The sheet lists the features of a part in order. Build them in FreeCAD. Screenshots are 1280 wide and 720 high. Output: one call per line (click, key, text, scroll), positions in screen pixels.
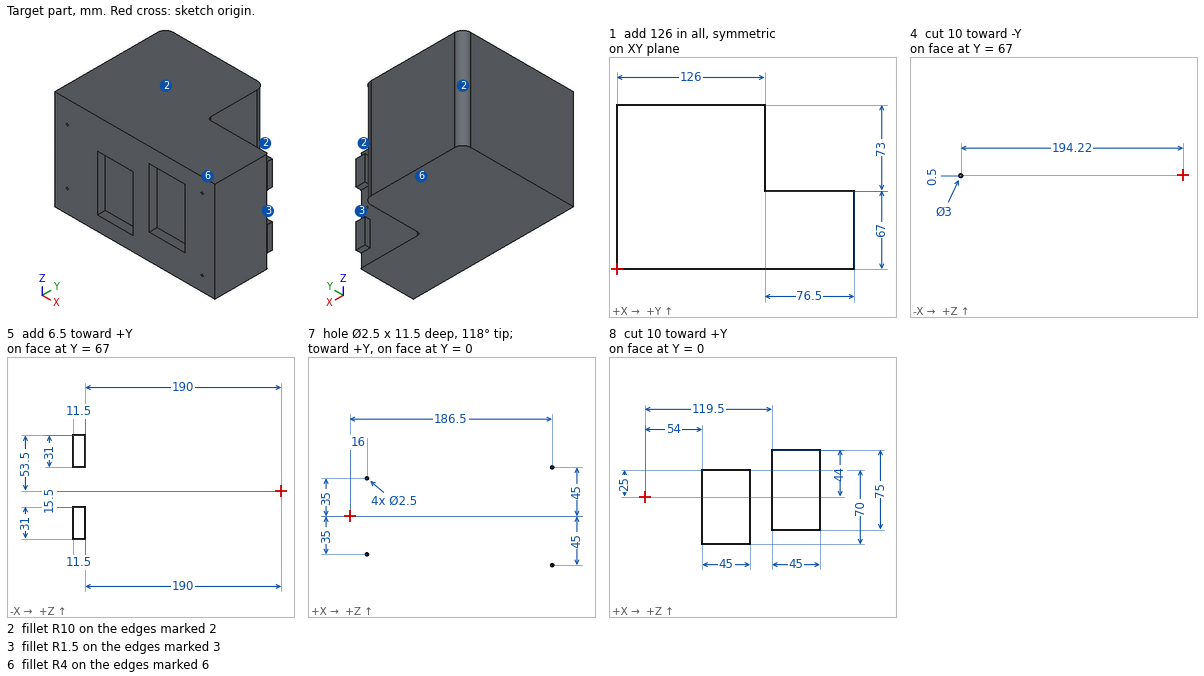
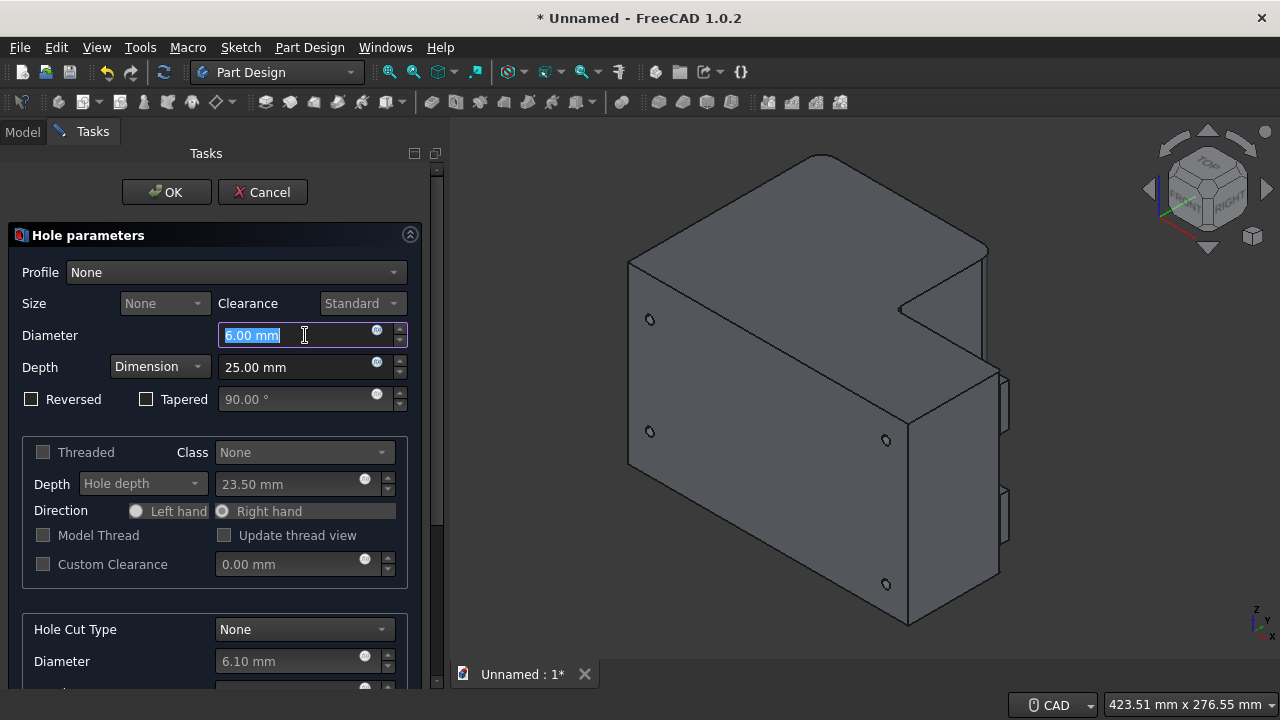
text(2.5)
key(Tab)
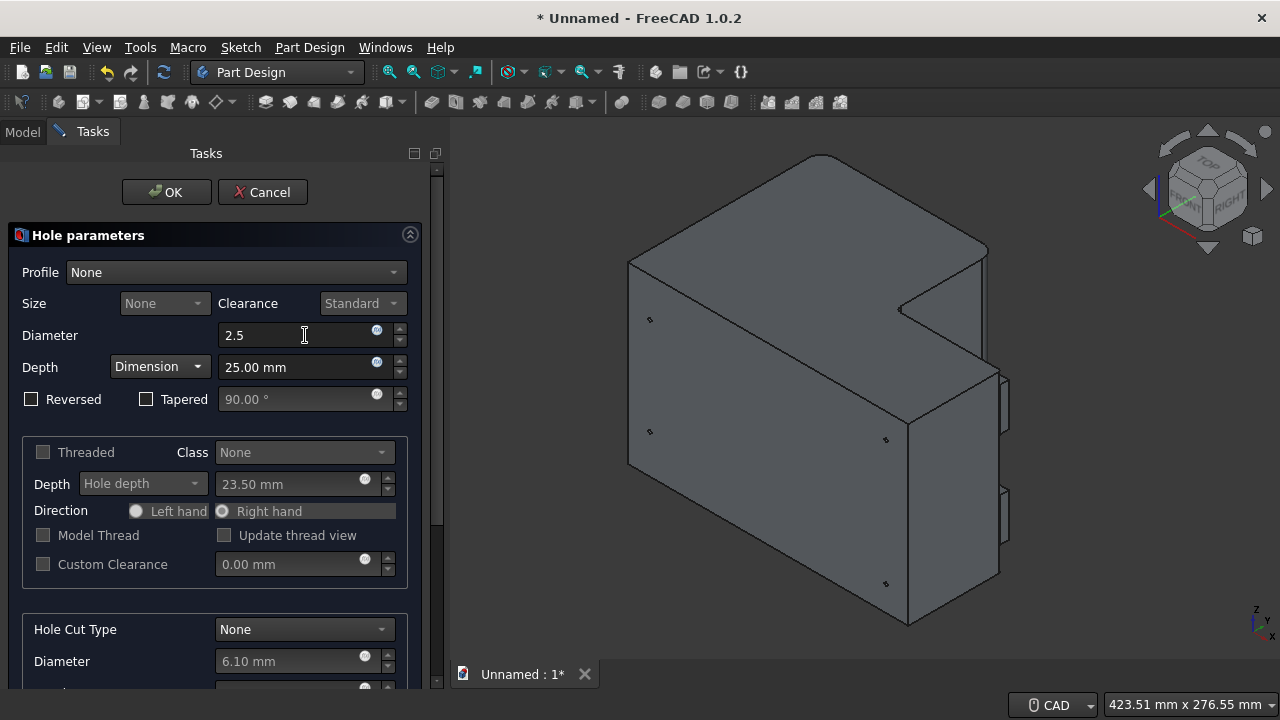
triple_click(305, 367)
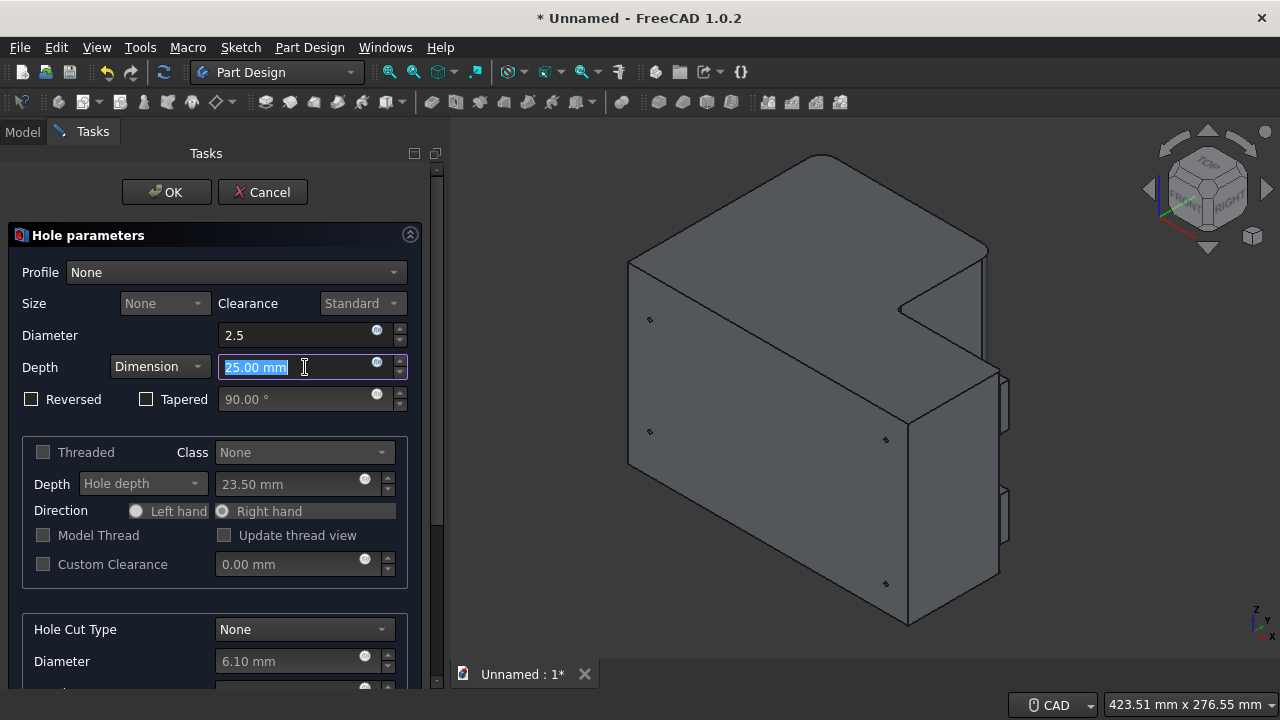
text(11.5)
key(Tab)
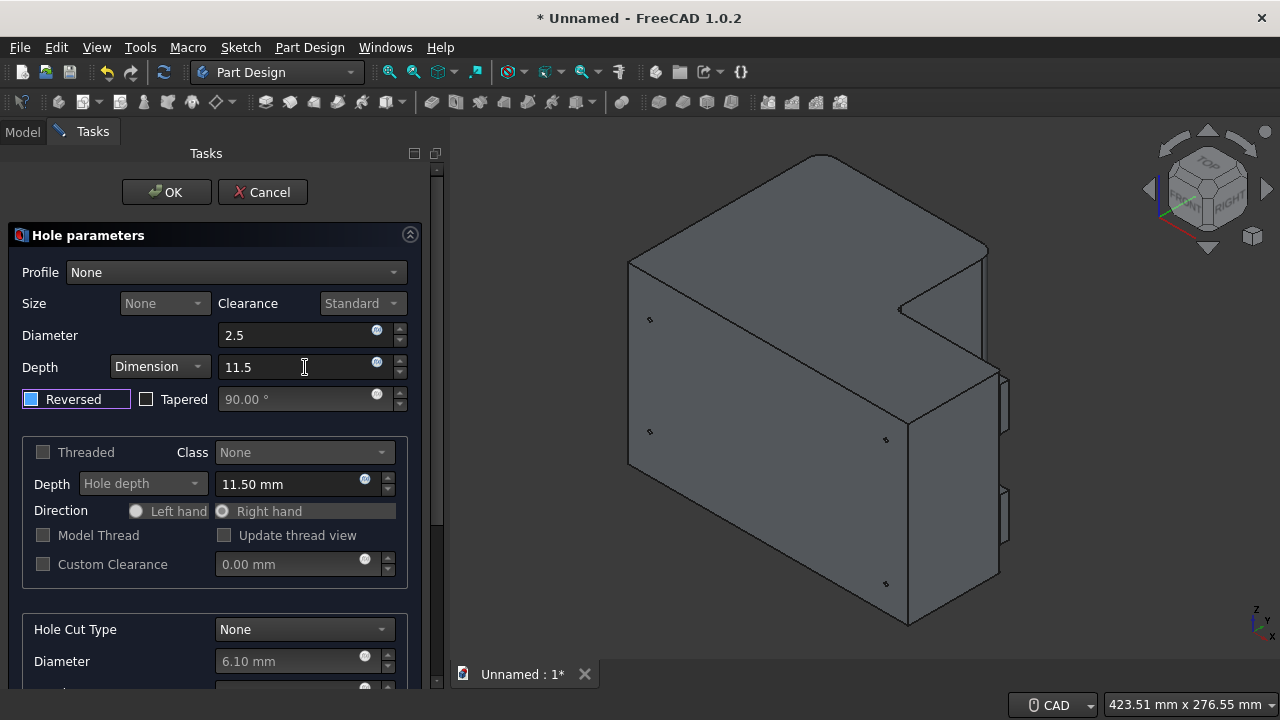
click(167, 192)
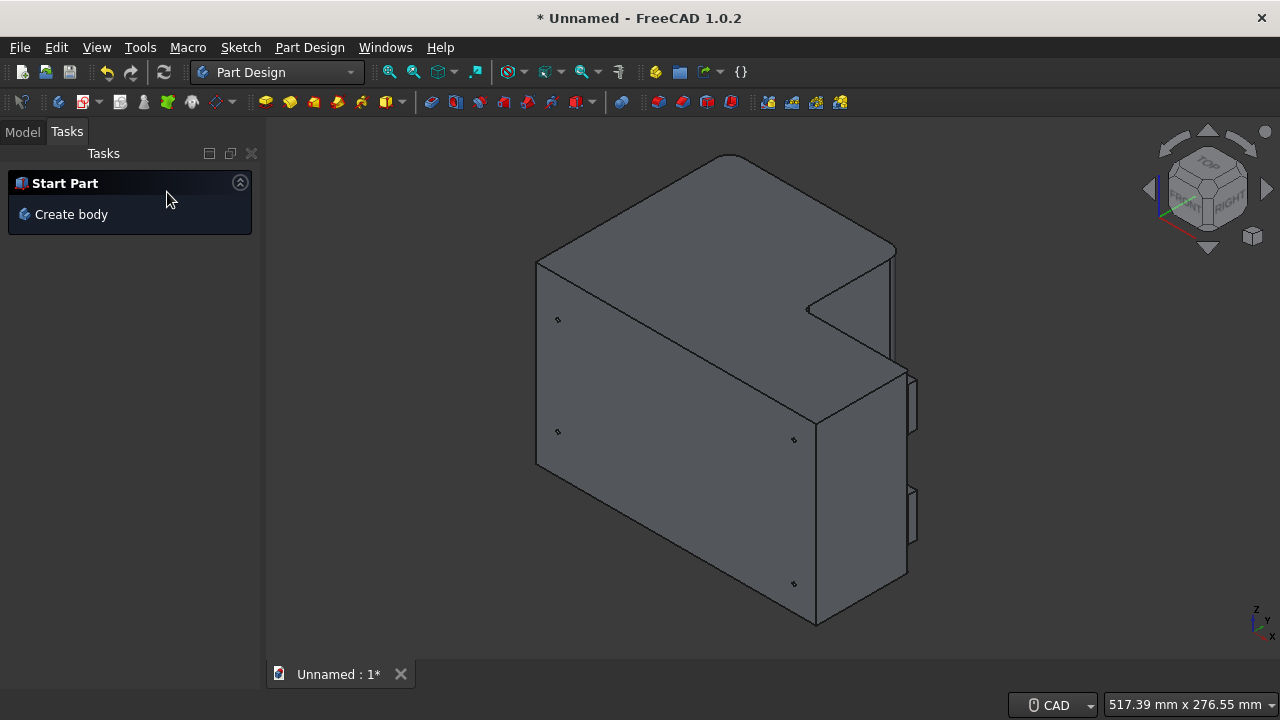
click(716, 466)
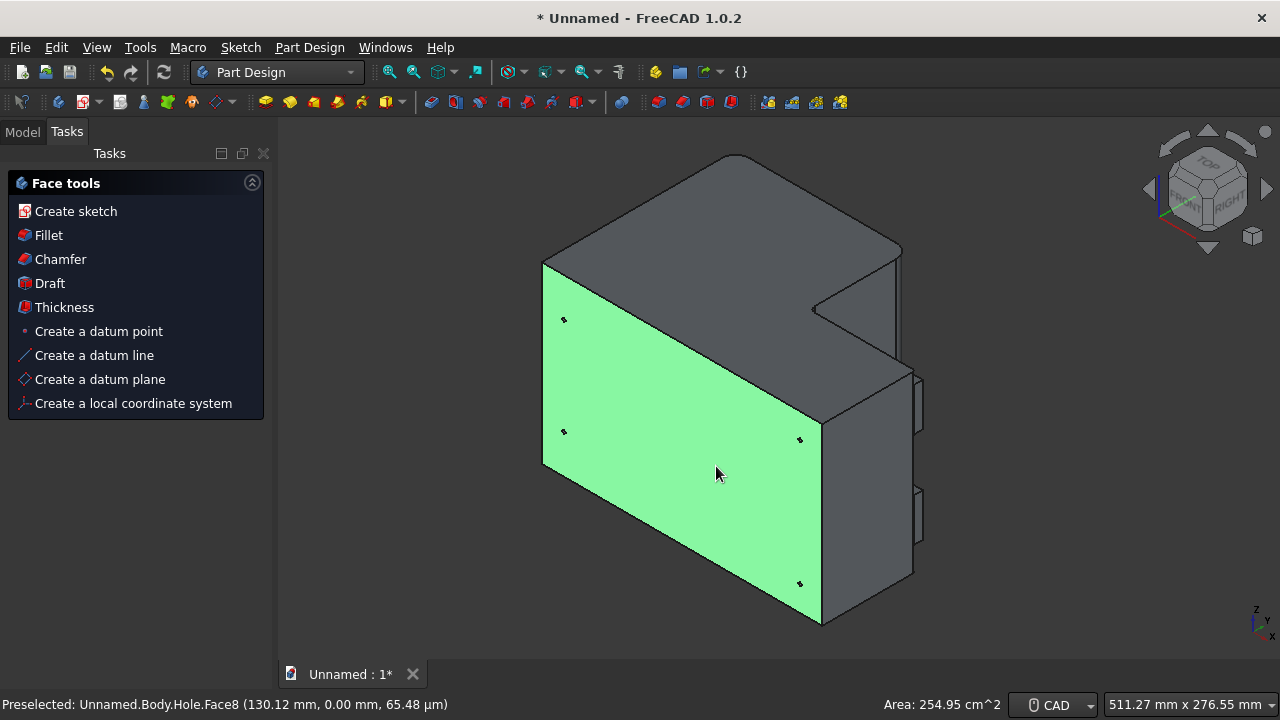
click(84, 102)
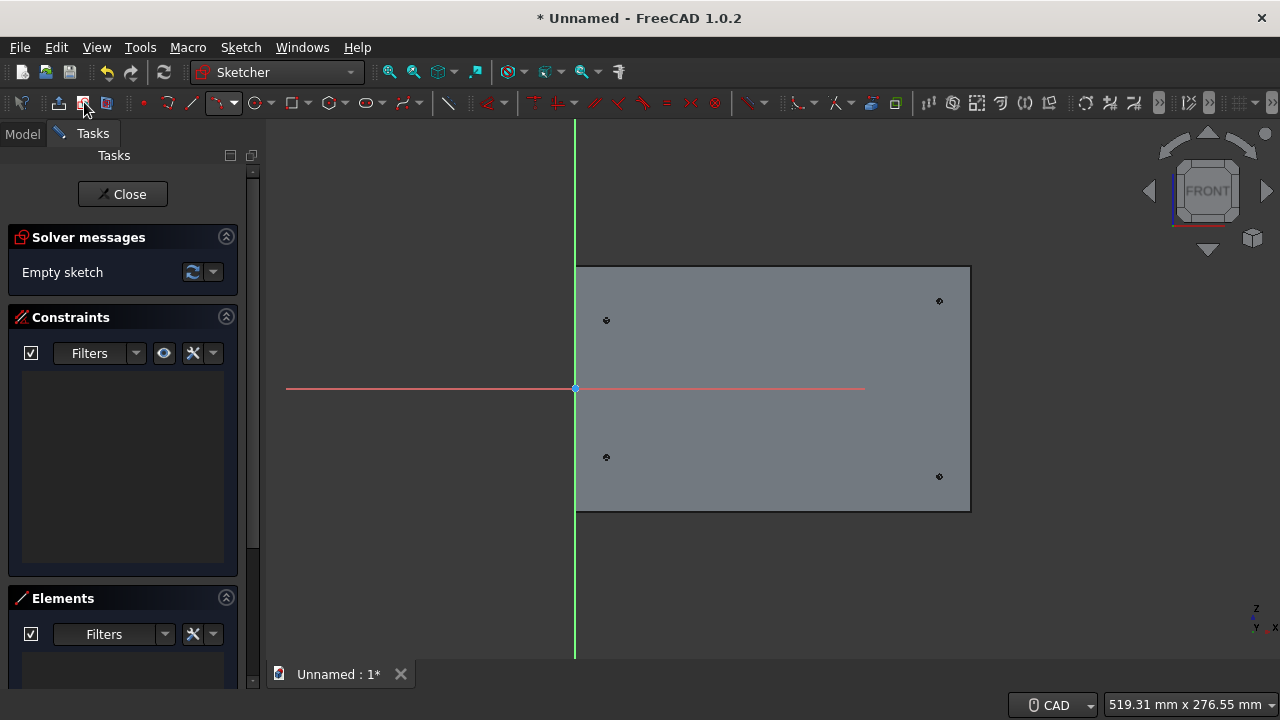
scroll(774, 391, up, 3)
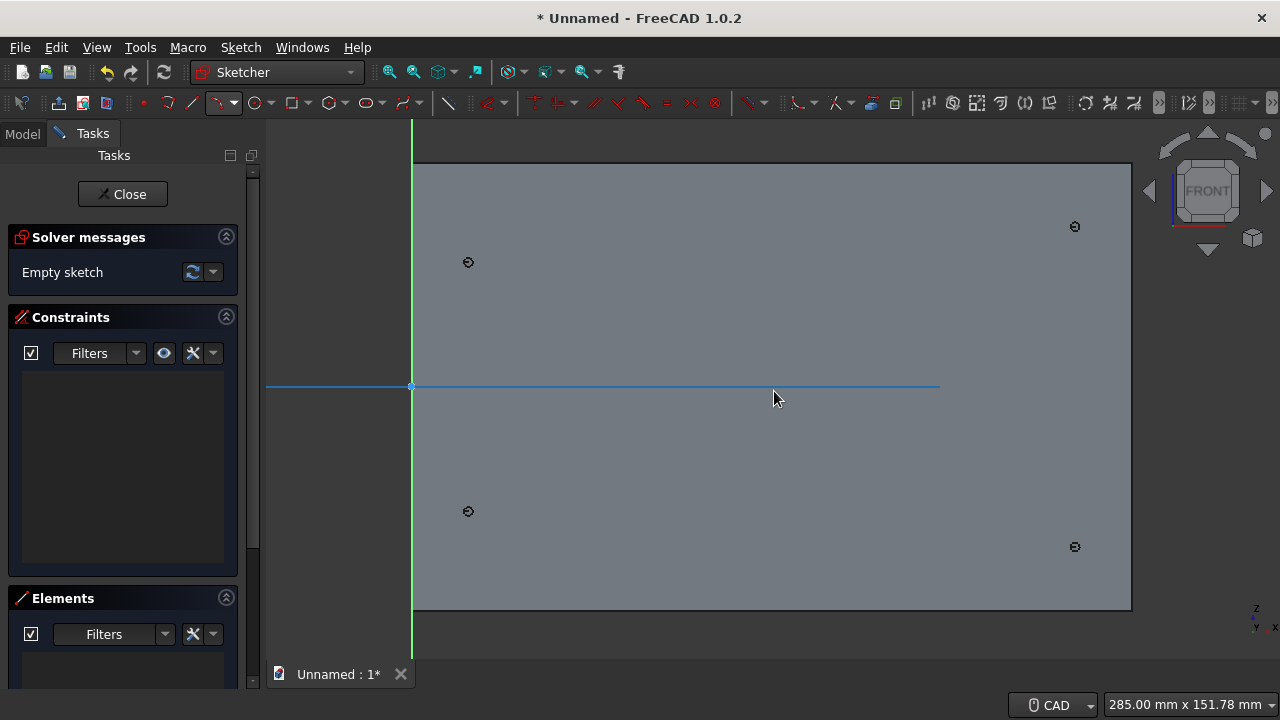
key(g)
key(r)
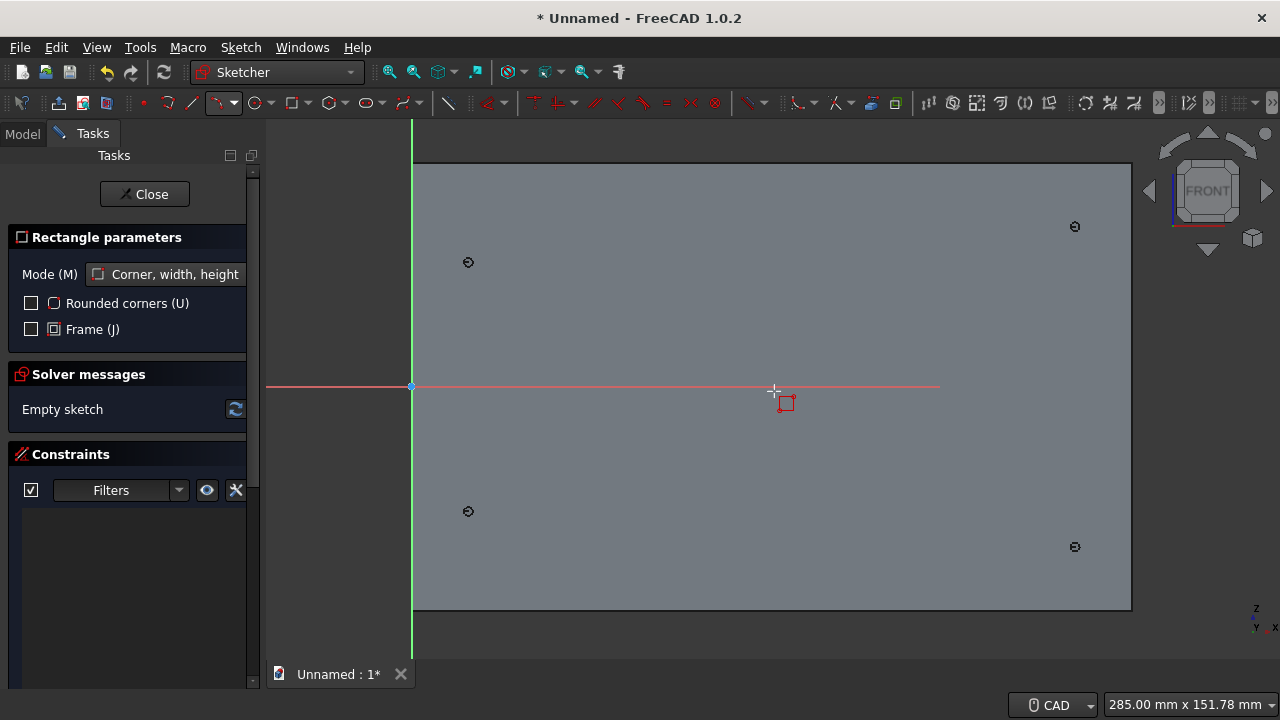
click(604, 298)
move(764, 547)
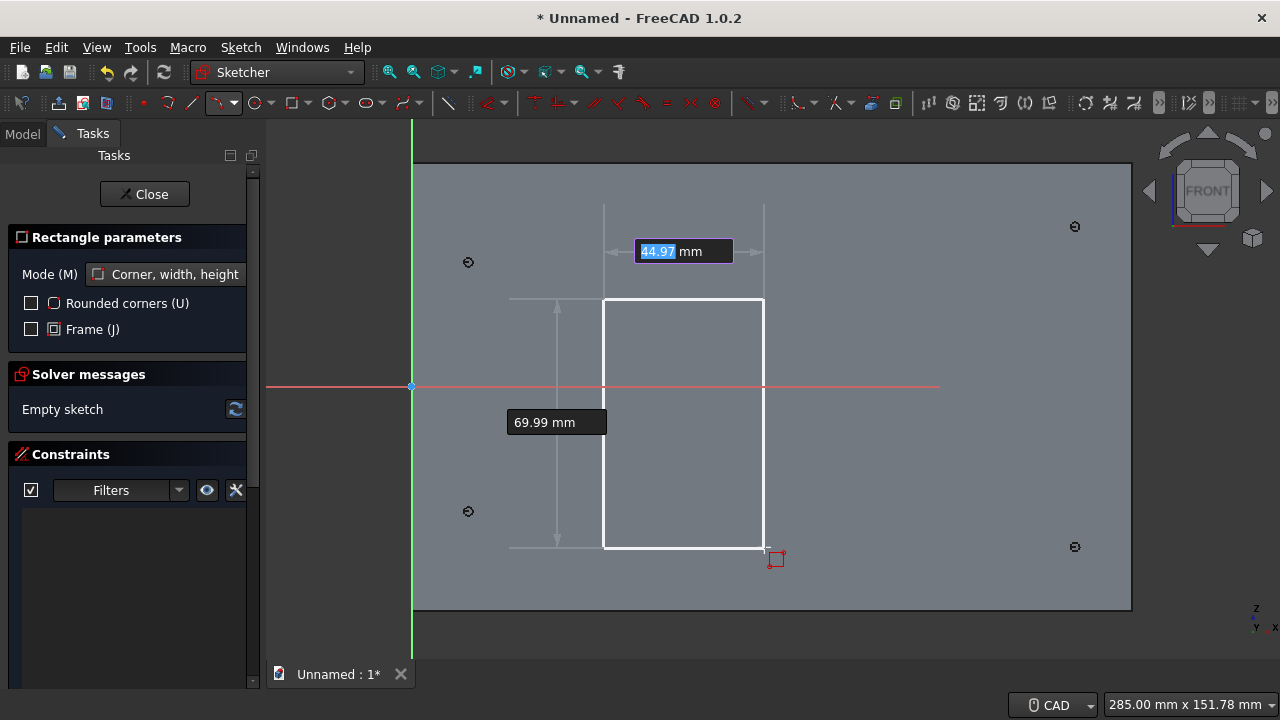
text(45)
key(Tab)
text(70)
key(Return)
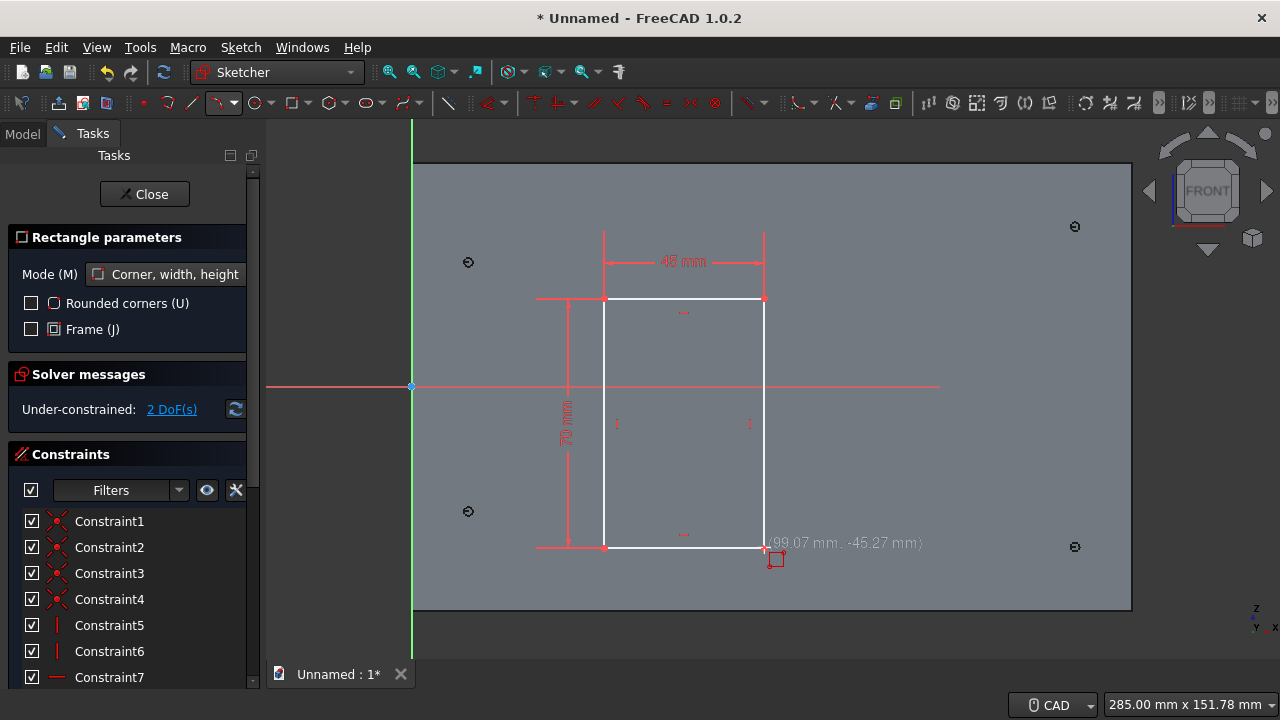
click(837, 230)
move(997, 497)